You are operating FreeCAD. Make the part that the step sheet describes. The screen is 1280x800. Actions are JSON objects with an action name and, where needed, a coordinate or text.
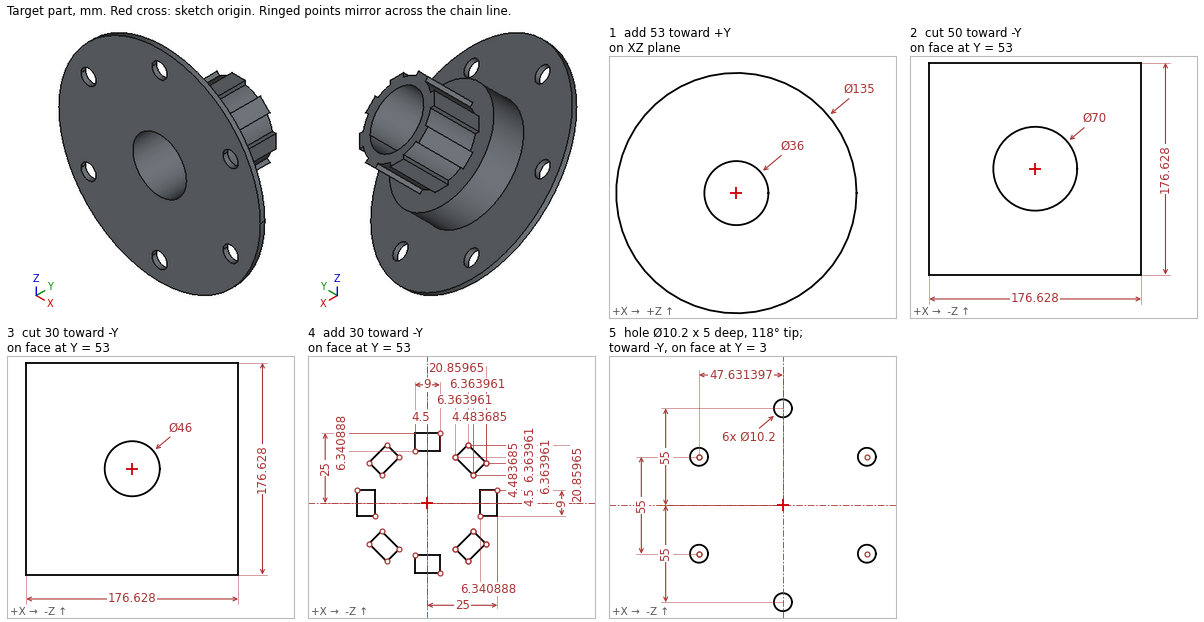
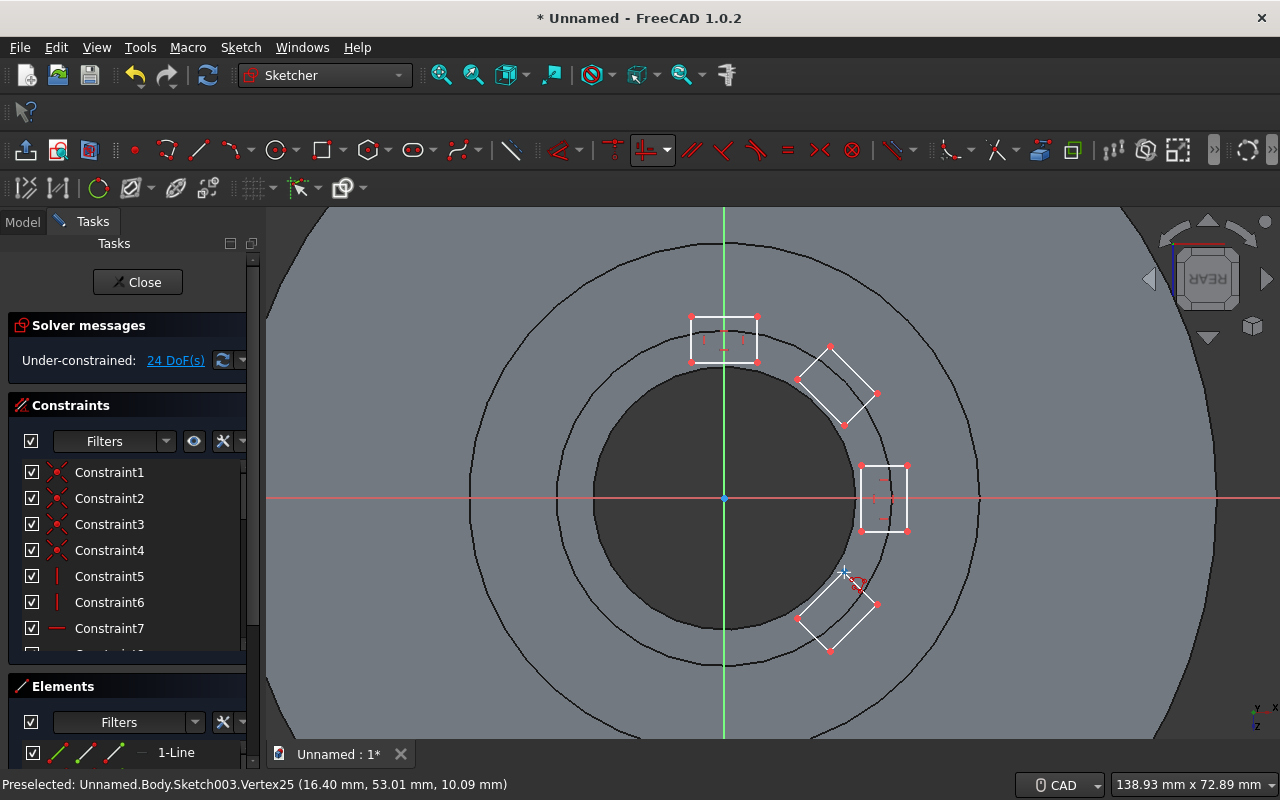
{"action": "left_click", "coordinate": [322, 150]}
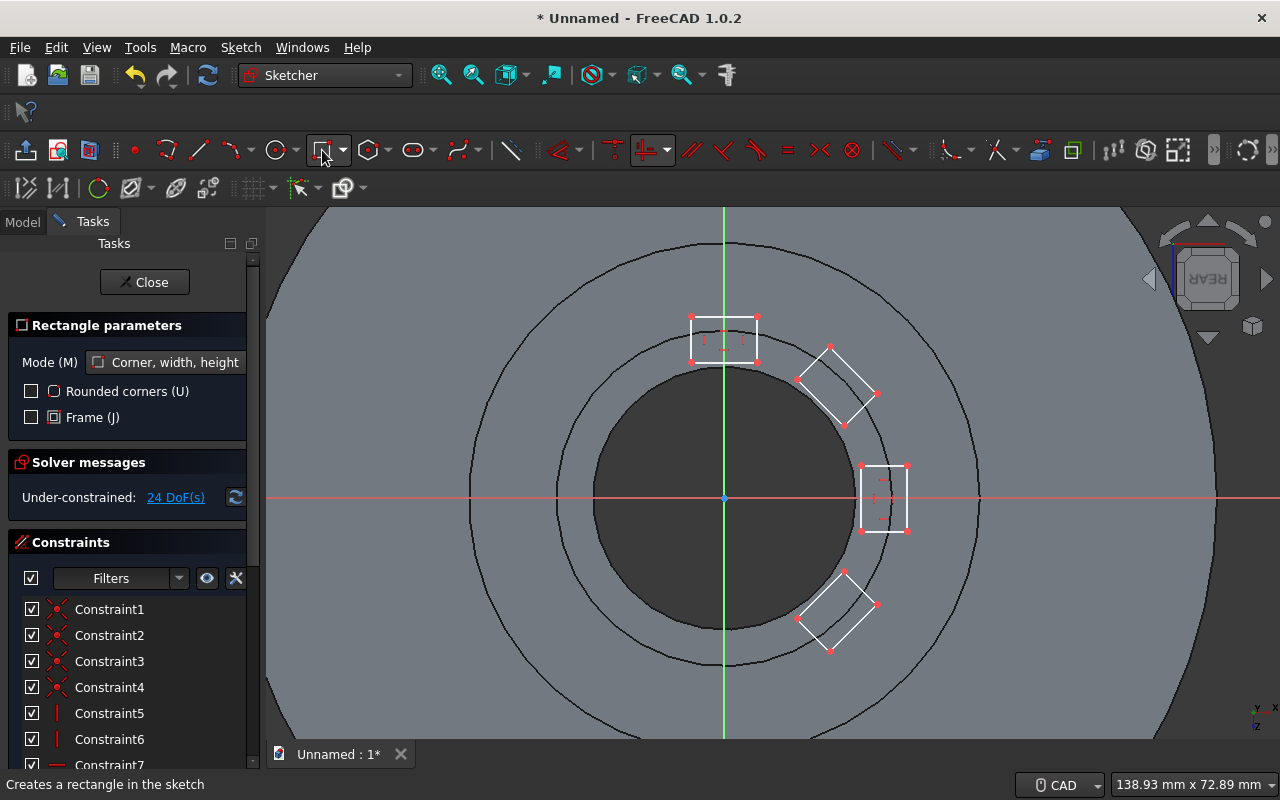
{"action": "left_click", "coordinate": [691, 635]}
{"action": "left_click", "coordinate": [757, 681]}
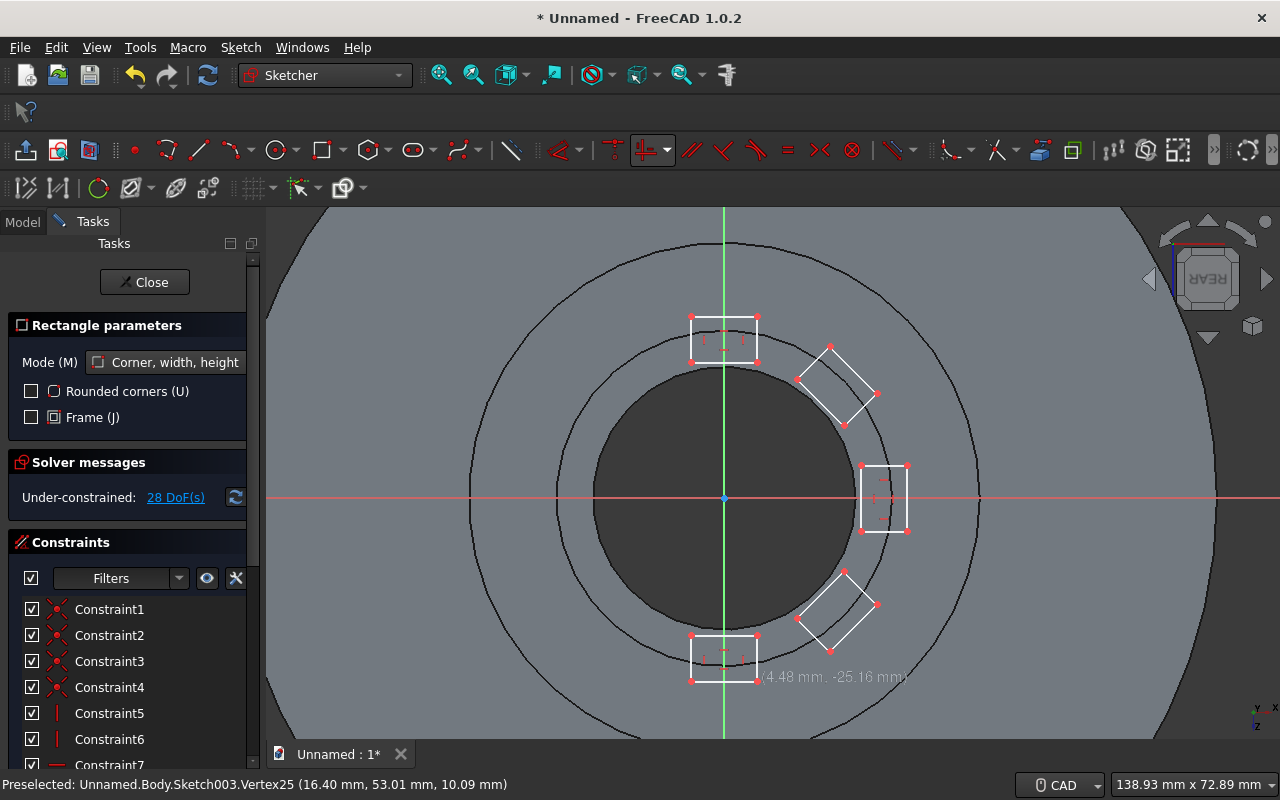
{"action": "left_click", "coordinate": [168, 150]}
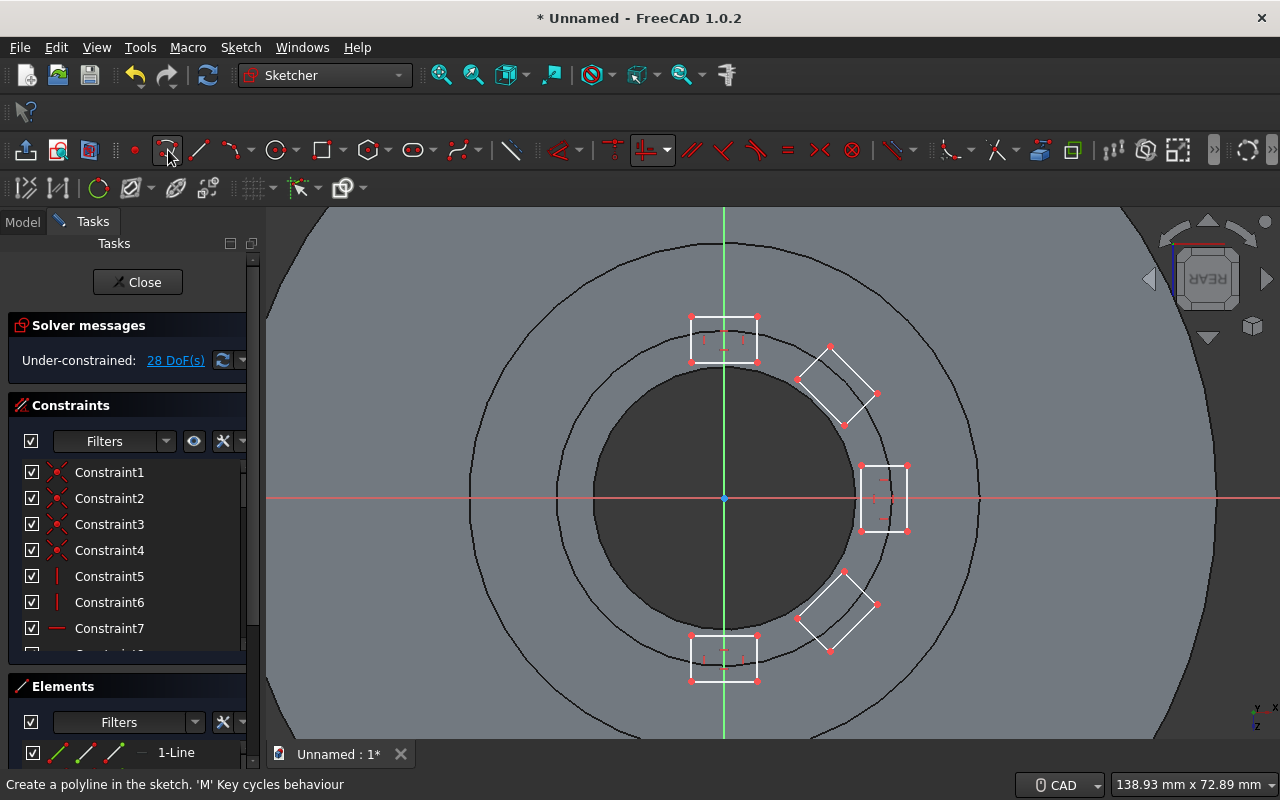
{"action": "left_click", "coordinate": [651, 618]}
{"action": "left_click", "coordinate": [605, 571]}
{"action": "left_click", "coordinate": [572, 604]}
{"action": "left_click", "coordinate": [619, 651]}
{"action": "left_click", "coordinate": [651, 619]}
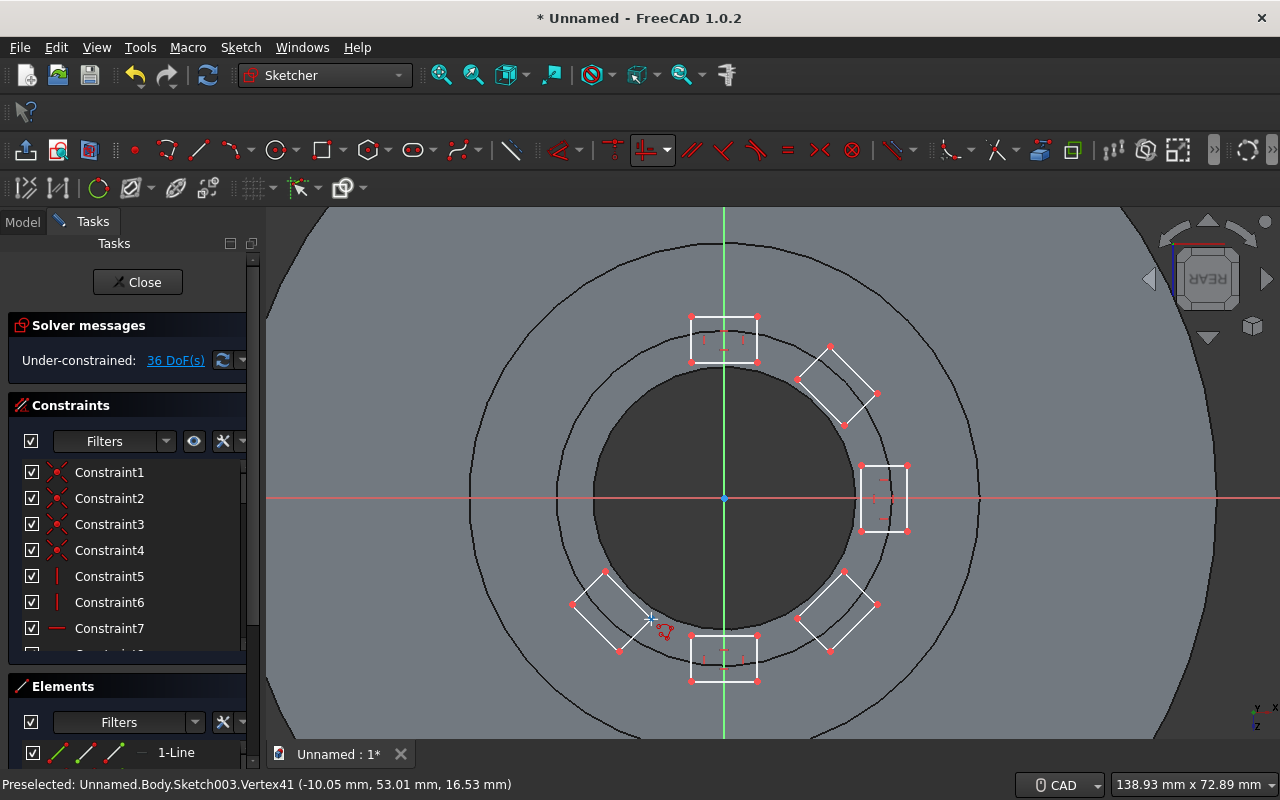
{"action": "left_click", "coordinate": [322, 150]}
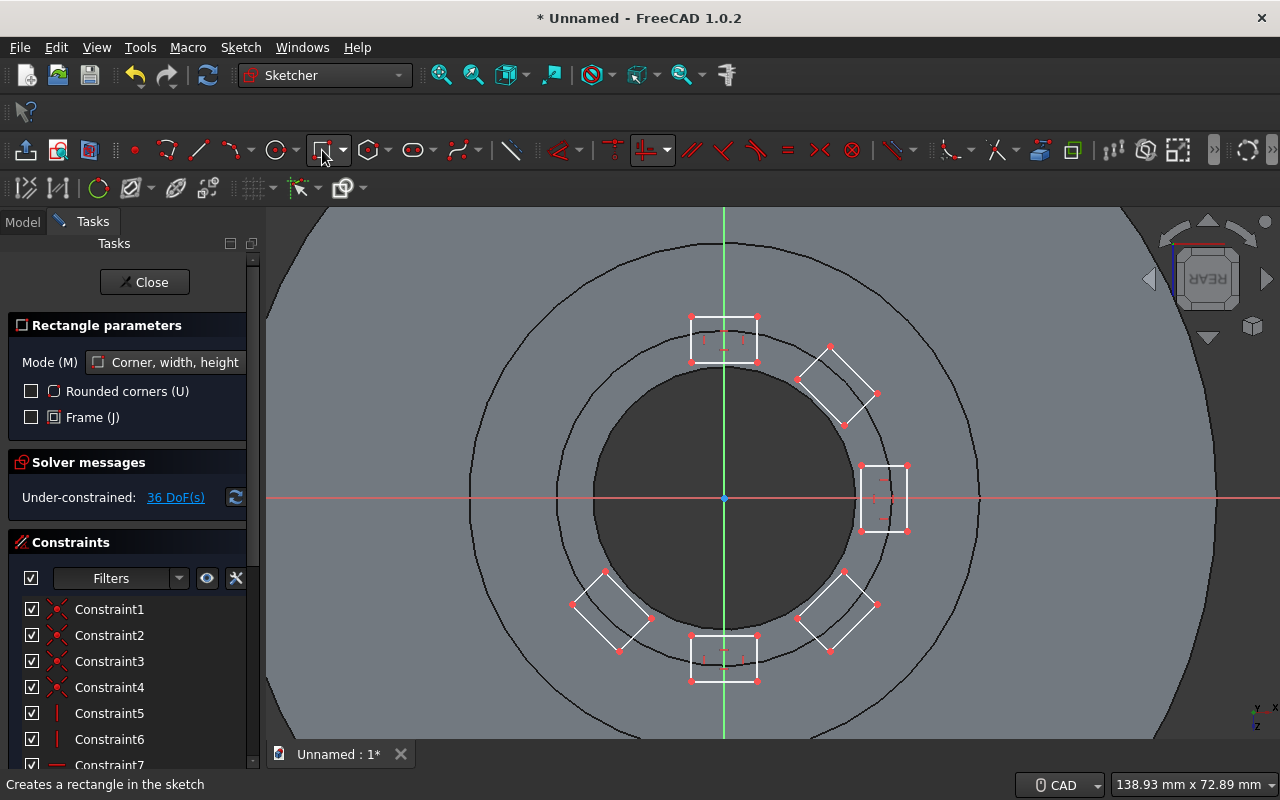
{"action": "left_click", "coordinate": [542, 465]}
{"action": "left_click", "coordinate": [588, 531]}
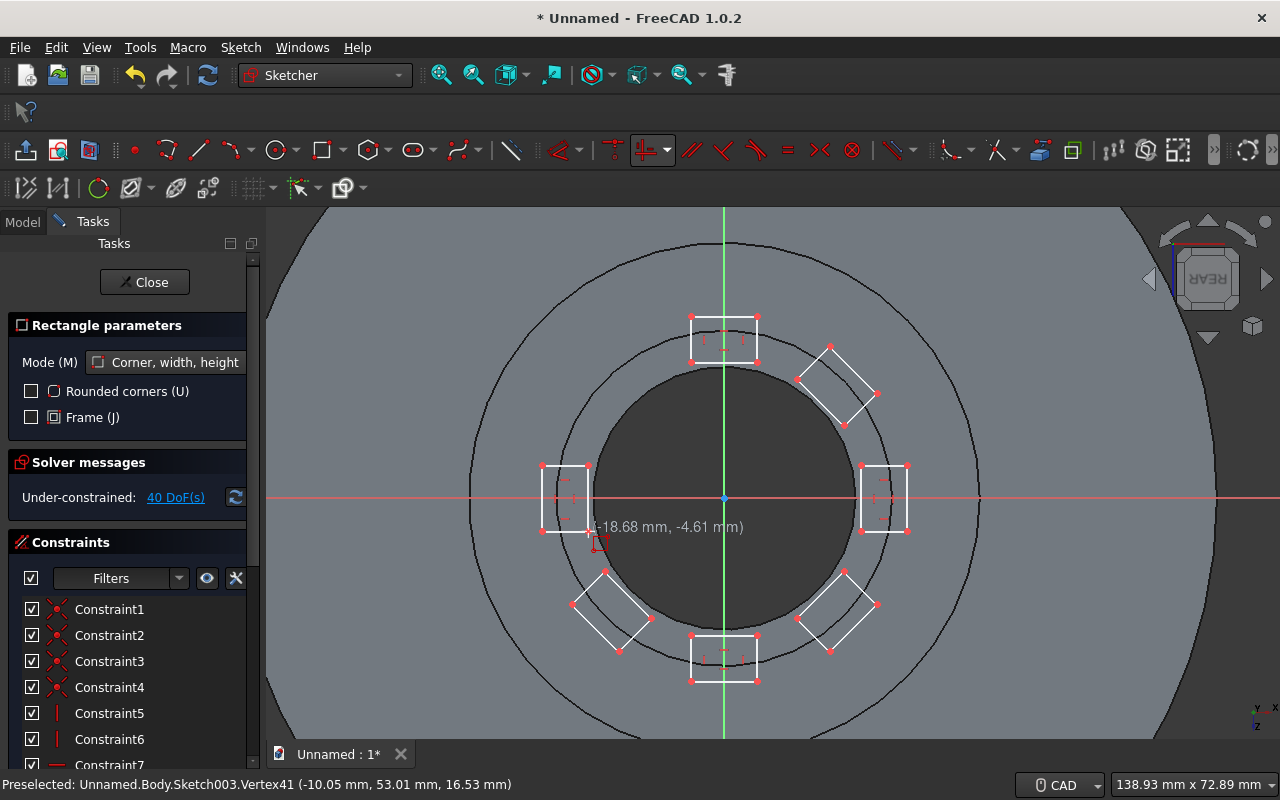
{"action": "left_click", "coordinate": [168, 150]}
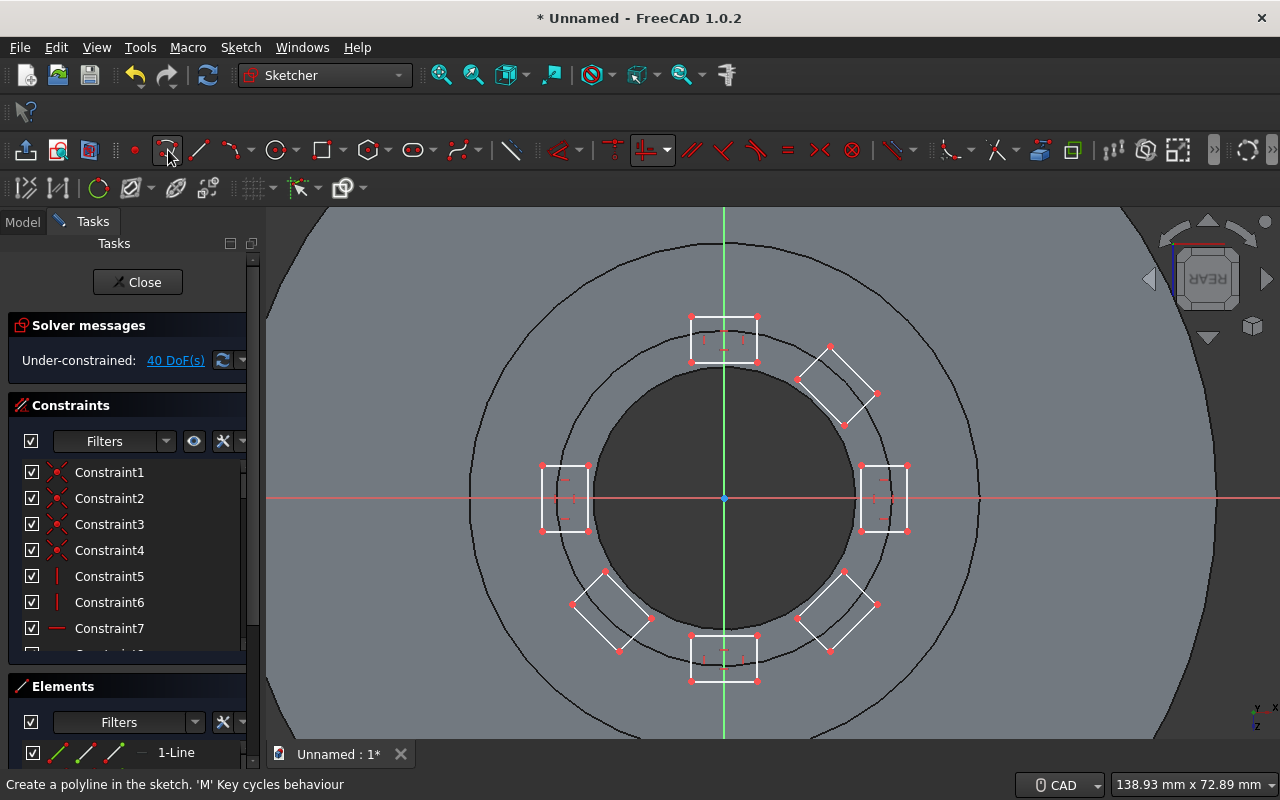
{"action": "left_click", "coordinate": [605, 425]}
{"action": "left_click", "coordinate": [651, 379]}
{"action": "left_click", "coordinate": [619, 346]}
{"action": "left_click", "coordinate": [572, 393]}
{"action": "left_click", "coordinate": [605, 426]}
{"action": "key", "text": "Escape"}
{"action": "key", "text": "Escape"}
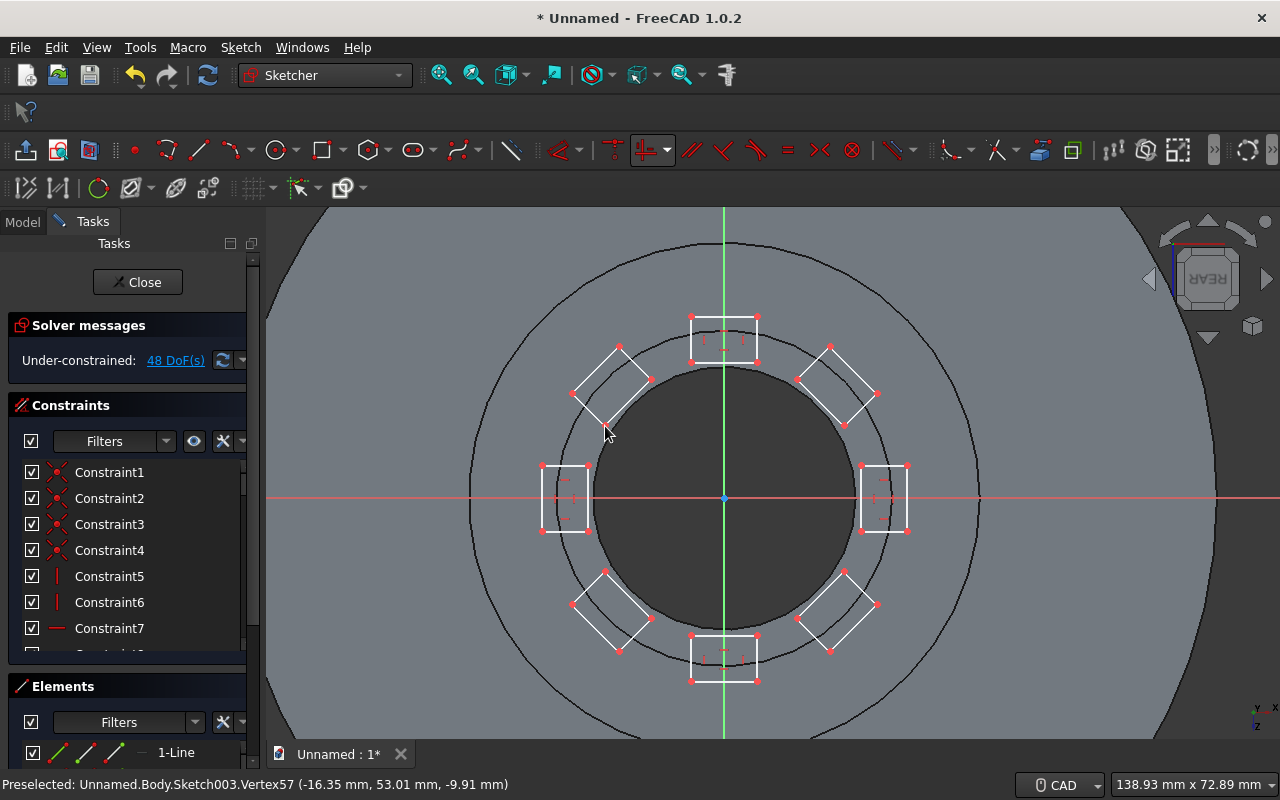
{"action": "left_click", "coordinate": [844, 426]}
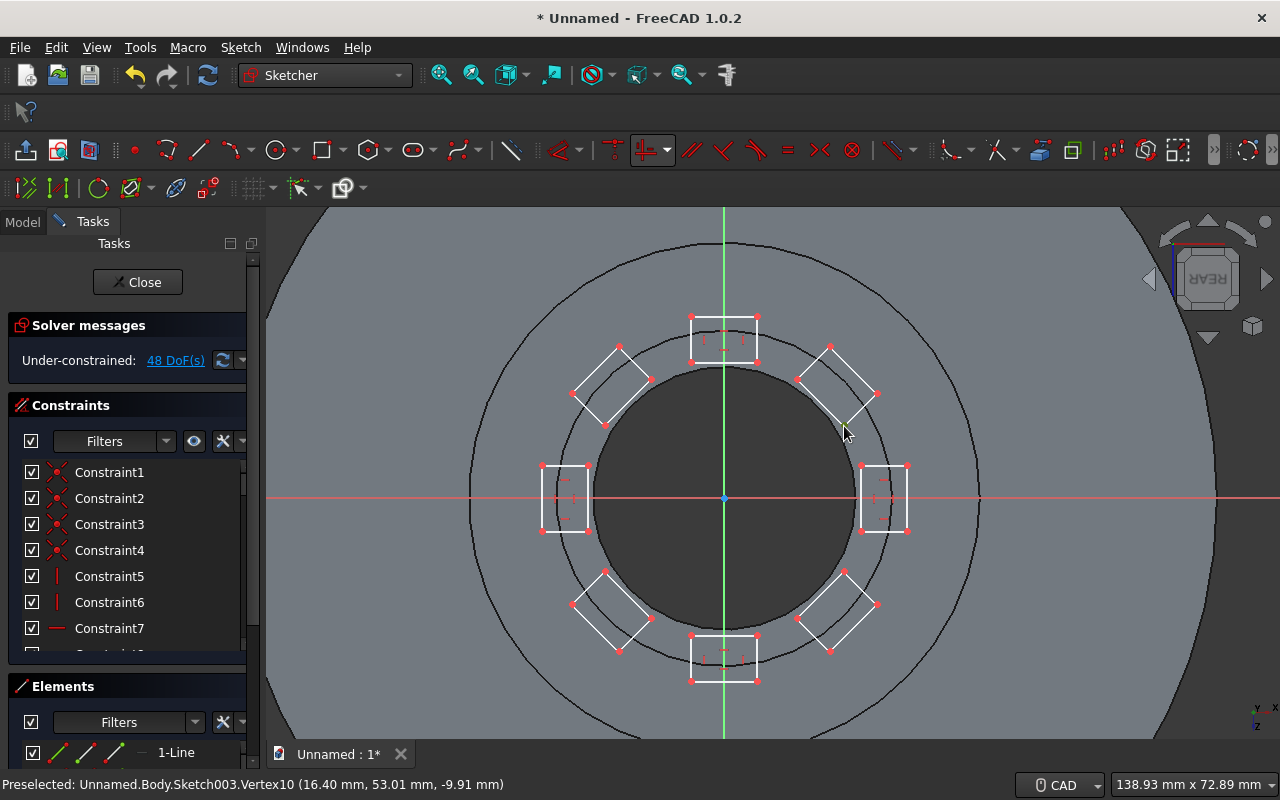
{"action": "left_click", "coordinate": [844, 572]}